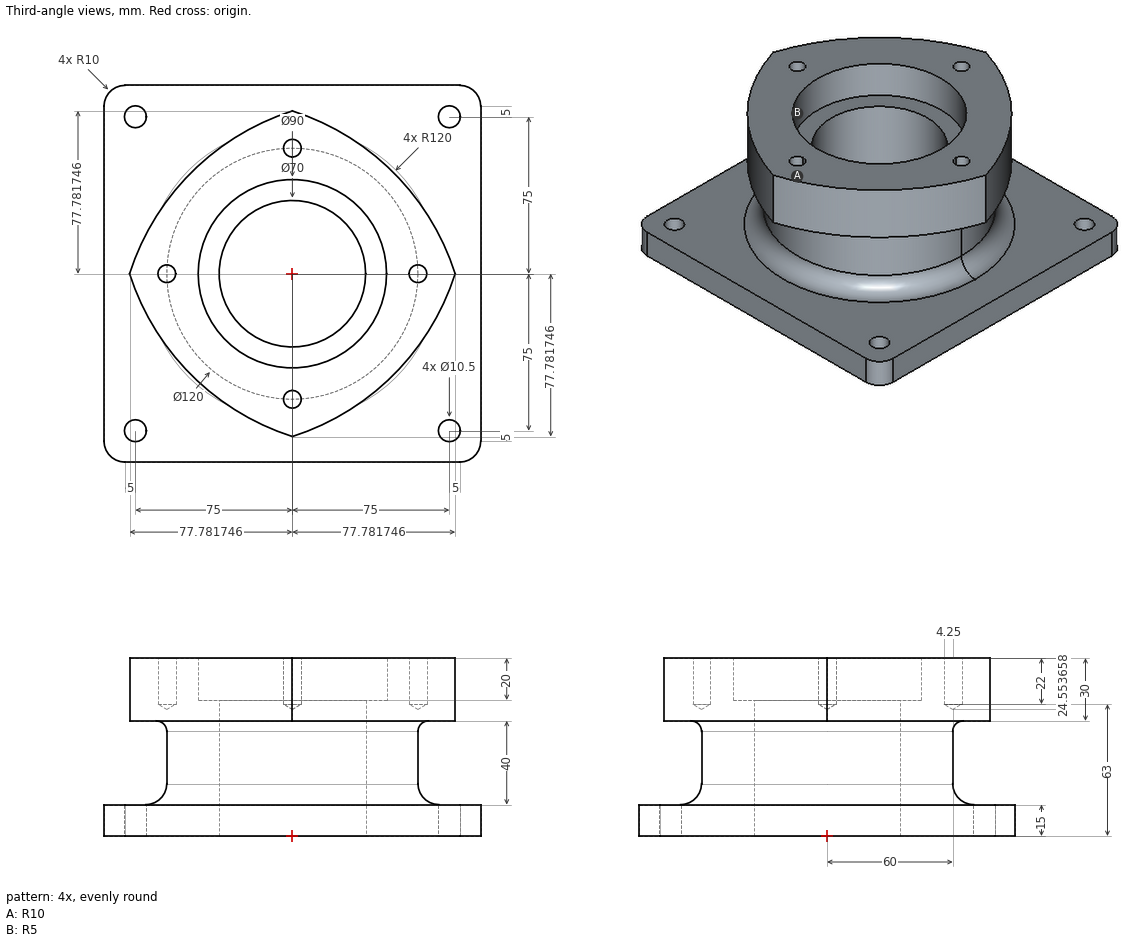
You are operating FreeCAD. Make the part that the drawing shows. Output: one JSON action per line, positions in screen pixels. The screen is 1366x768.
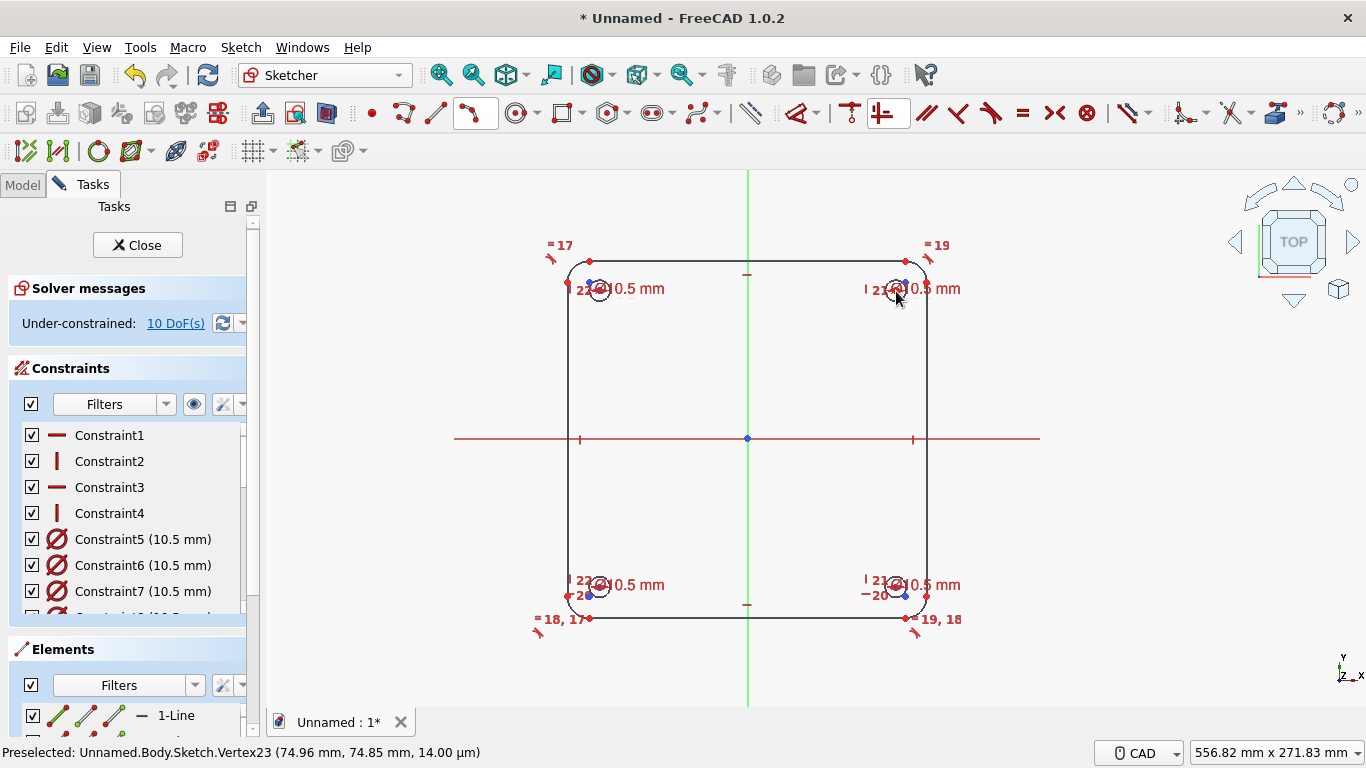
{"action": "left_click", "coordinate": [600, 291]}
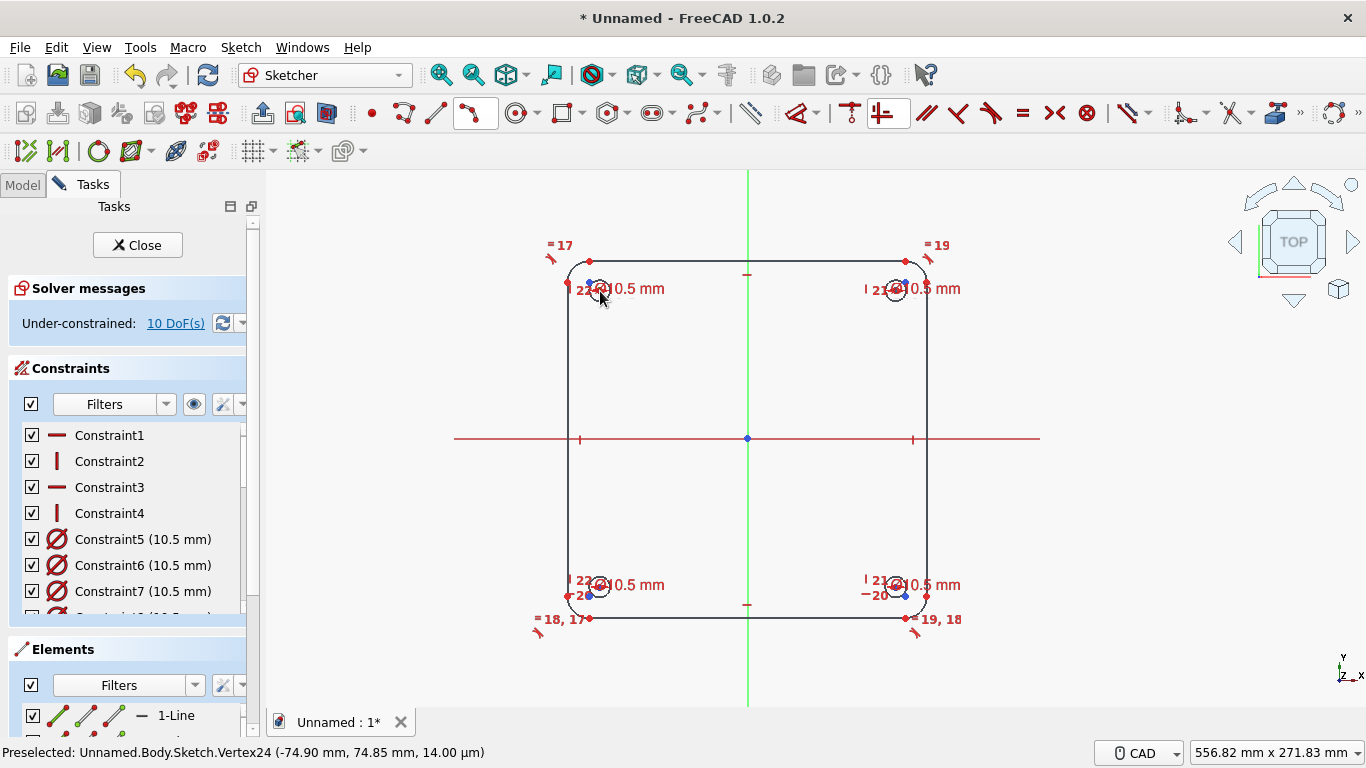
{"action": "left_click", "coordinate": [904, 114]}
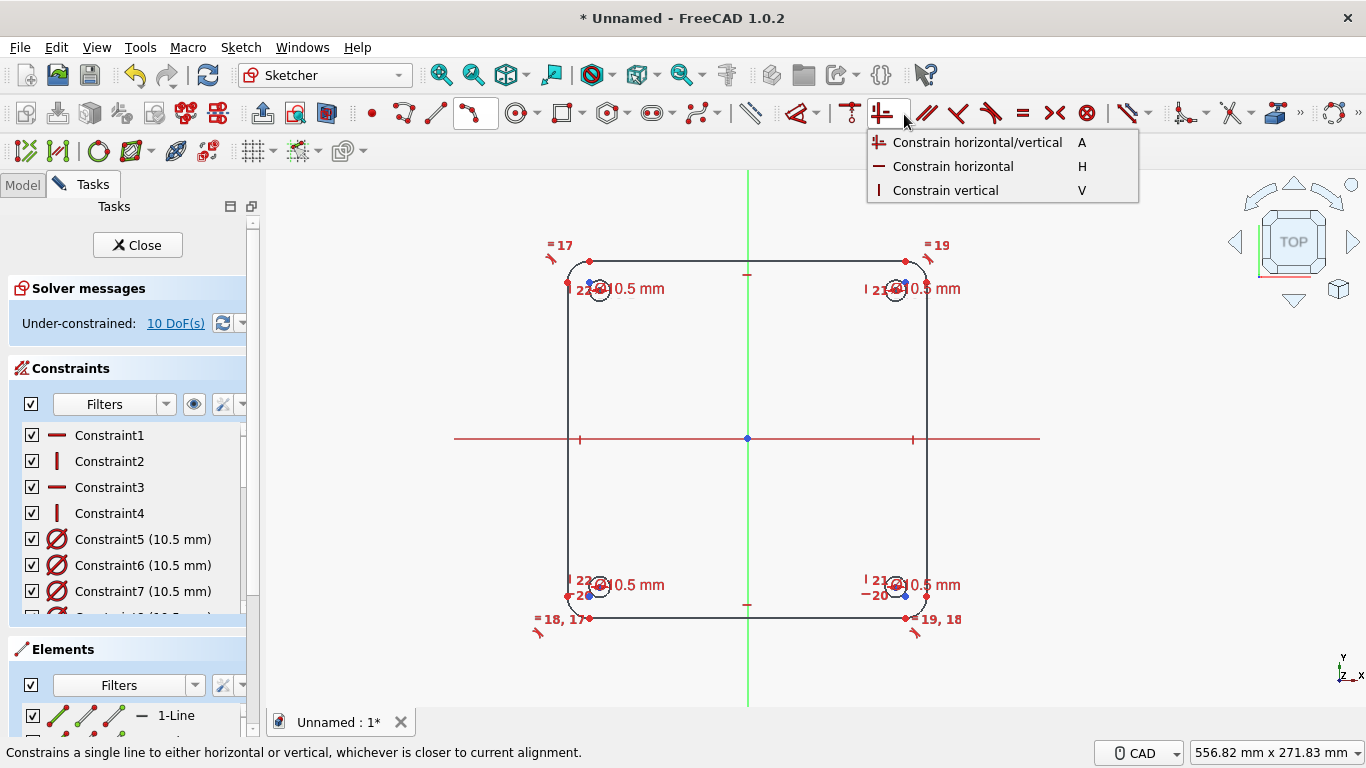
{"action": "left_click", "coordinate": [1003, 166]}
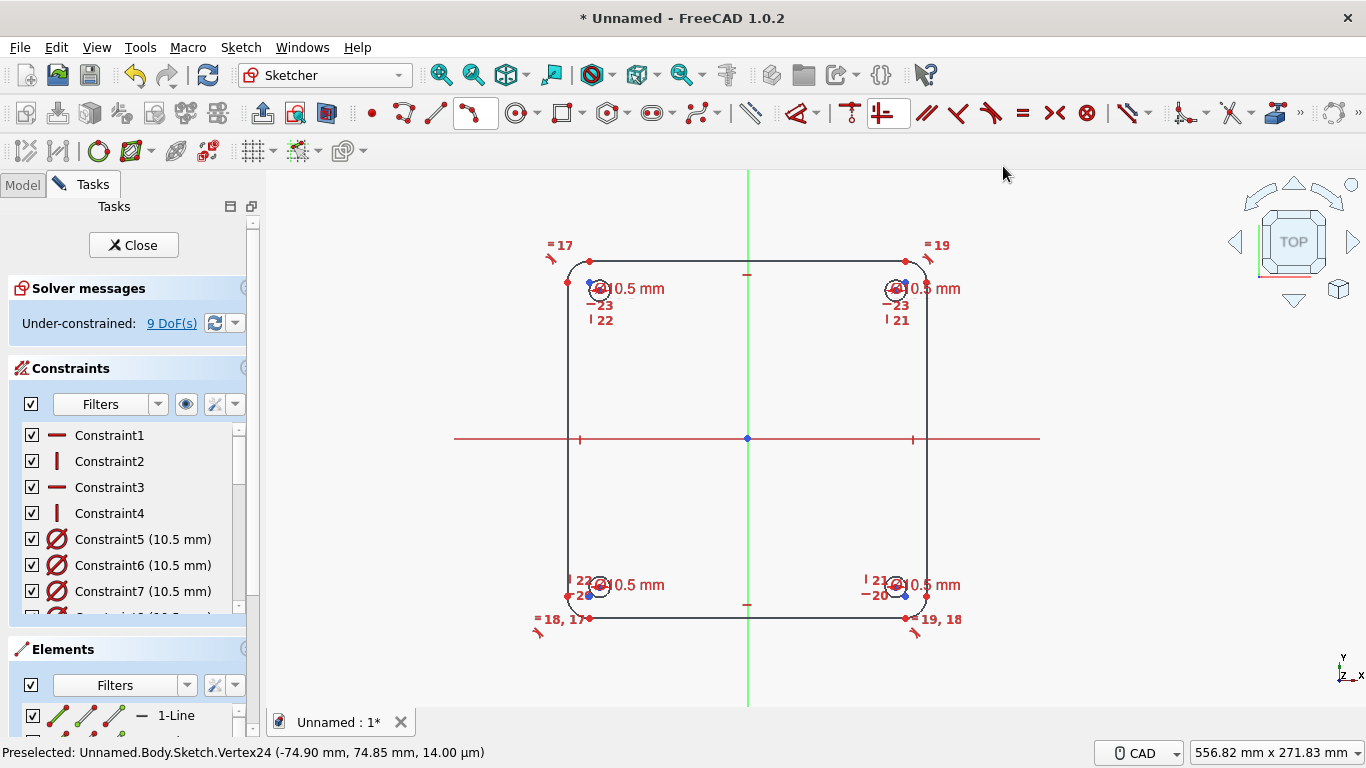
{"action": "left_click", "coordinate": [796, 114]}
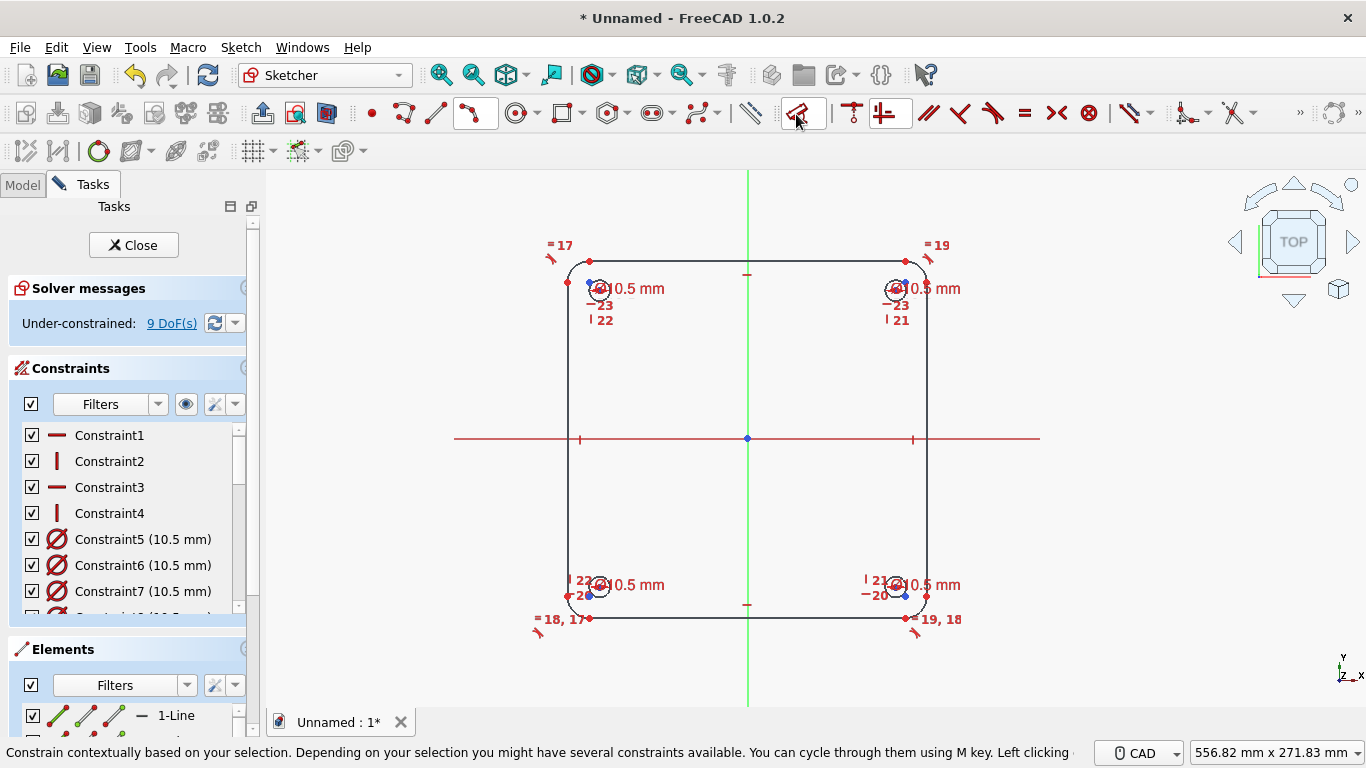
{"action": "scroll", "coordinate": [579, 264], "scroll_direction": "up", "scroll_amount": 4}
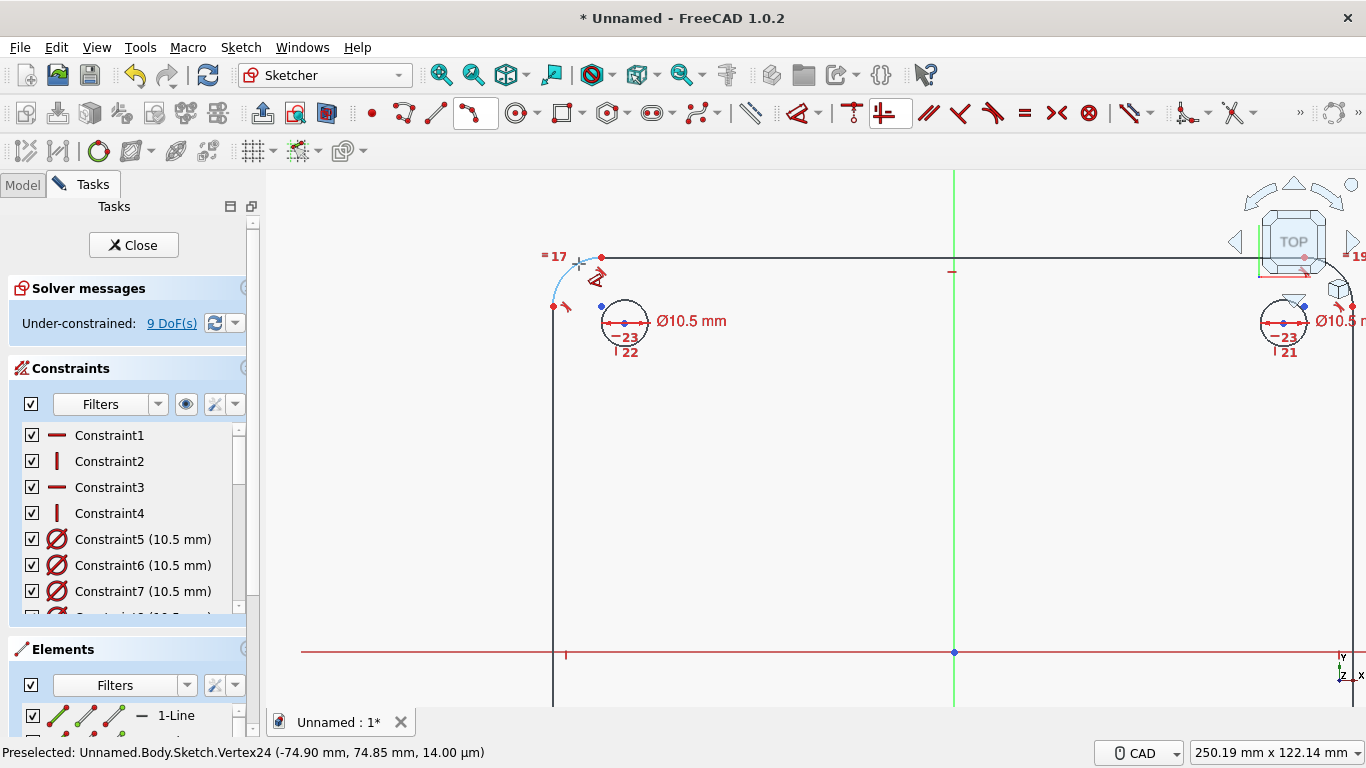
{"action": "left_click", "coordinate": [579, 263]}
{"action": "left_click", "coordinate": [564, 235]}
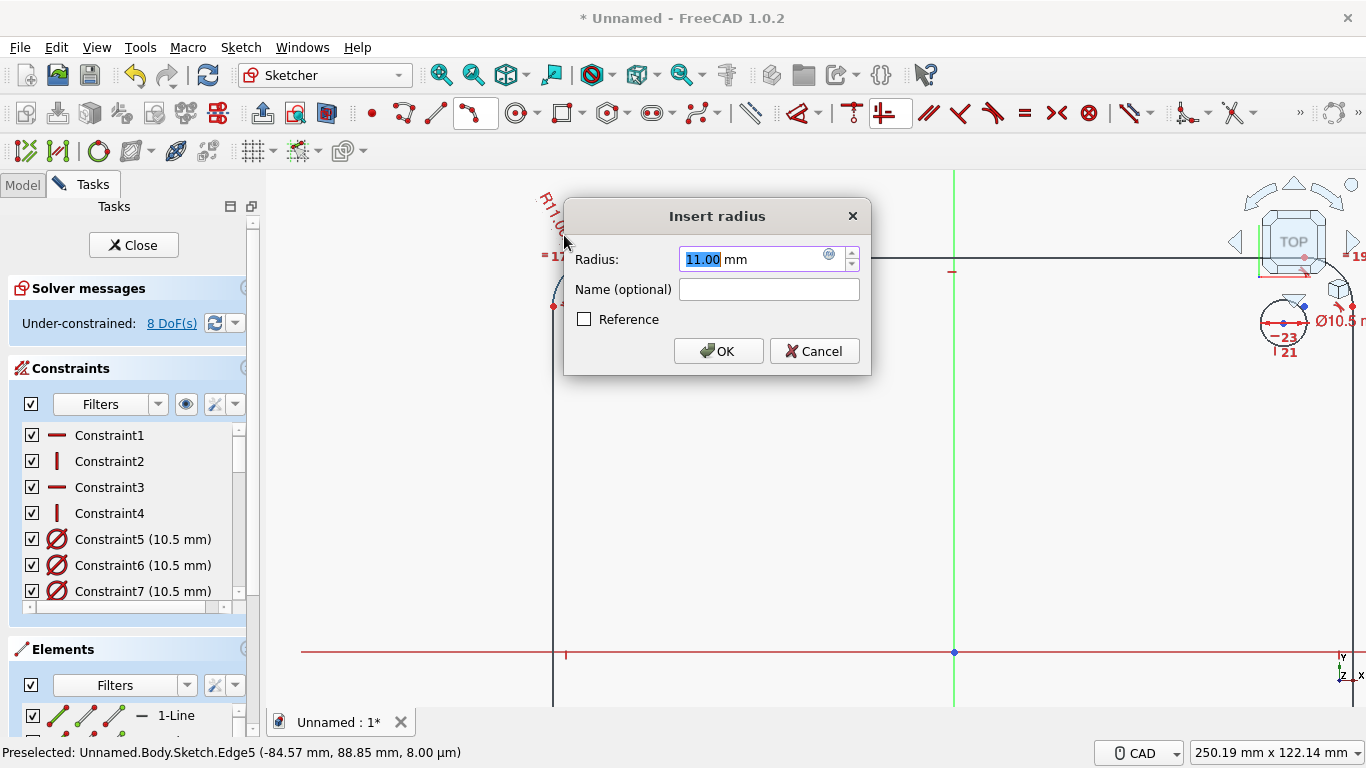
{"action": "type", "text": "10"}
{"action": "key", "text": "Return"}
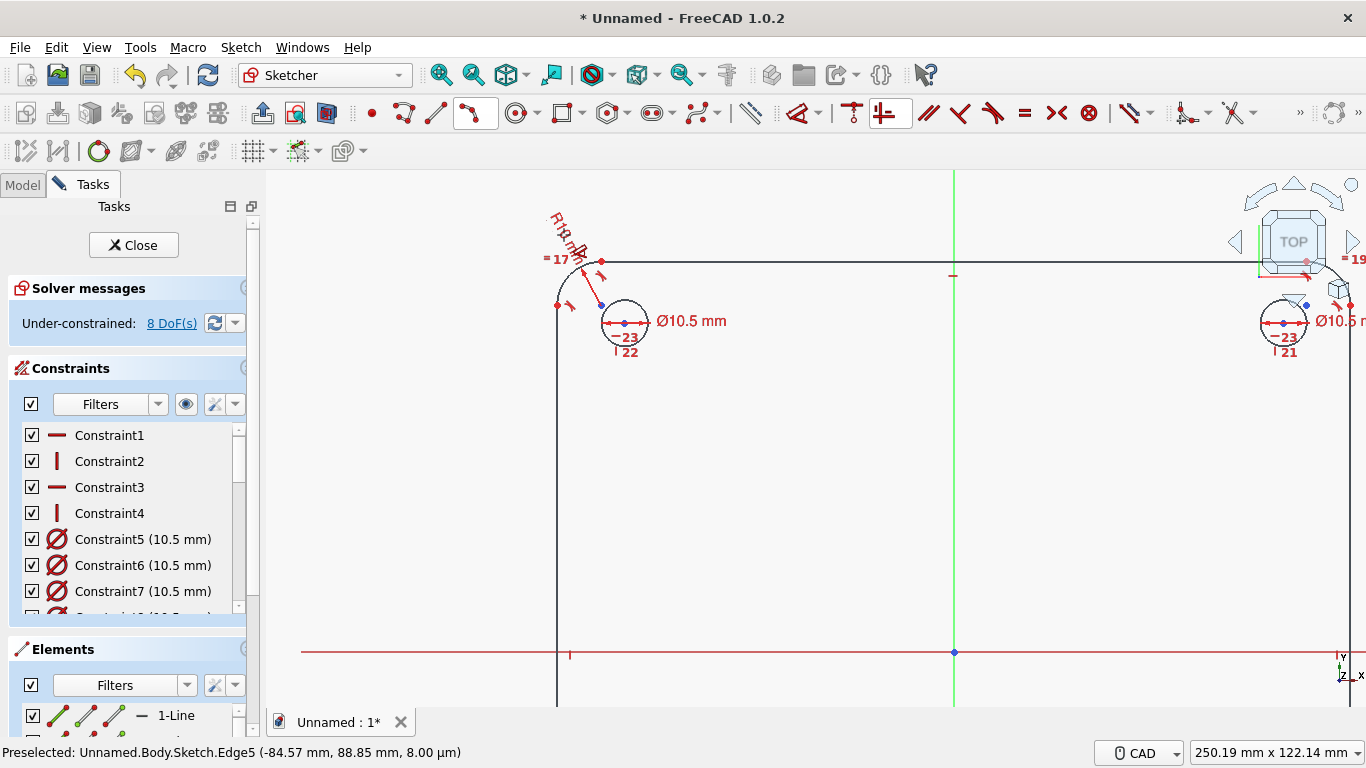
{"action": "scroll", "coordinate": [579, 264], "scroll_direction": "down", "scroll_amount": 4}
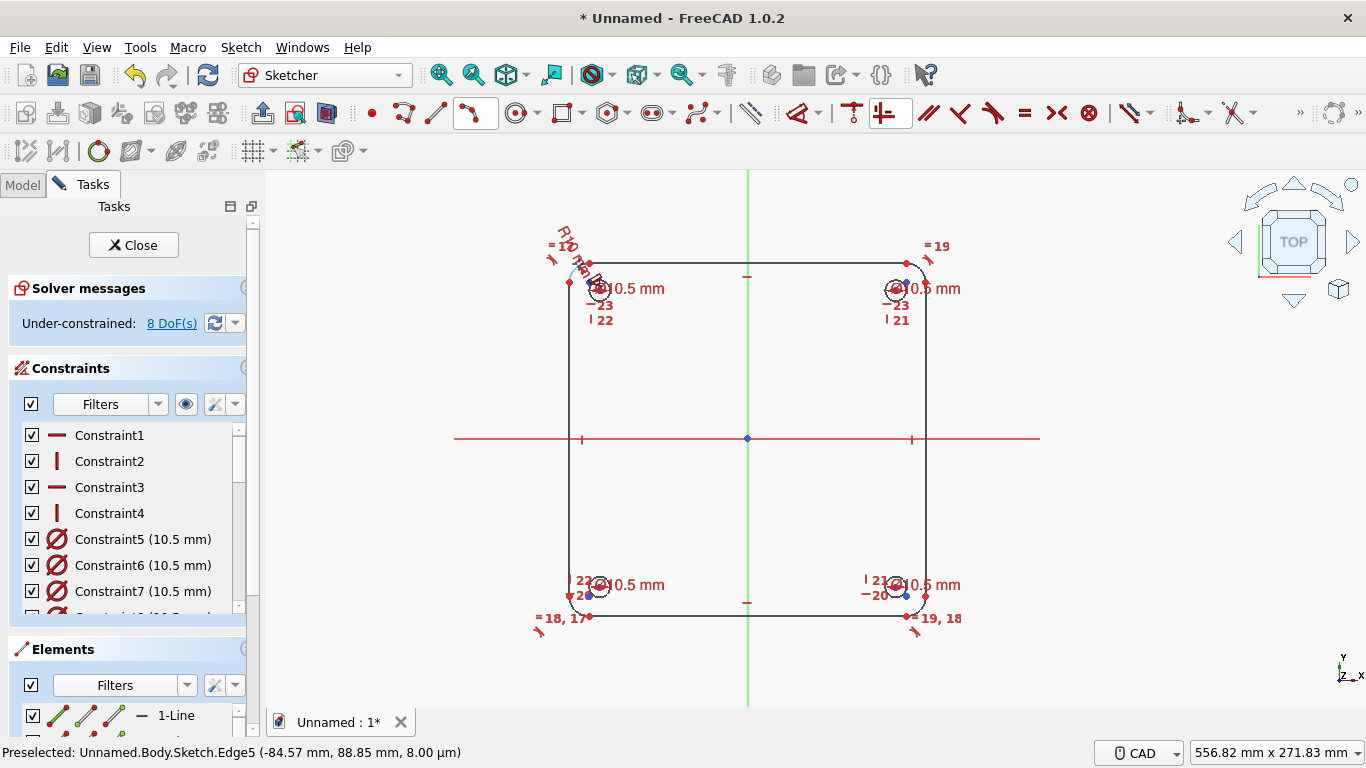
{"action": "left_click", "coordinate": [896, 587]}
{"action": "left_click", "coordinate": [822, 405]}